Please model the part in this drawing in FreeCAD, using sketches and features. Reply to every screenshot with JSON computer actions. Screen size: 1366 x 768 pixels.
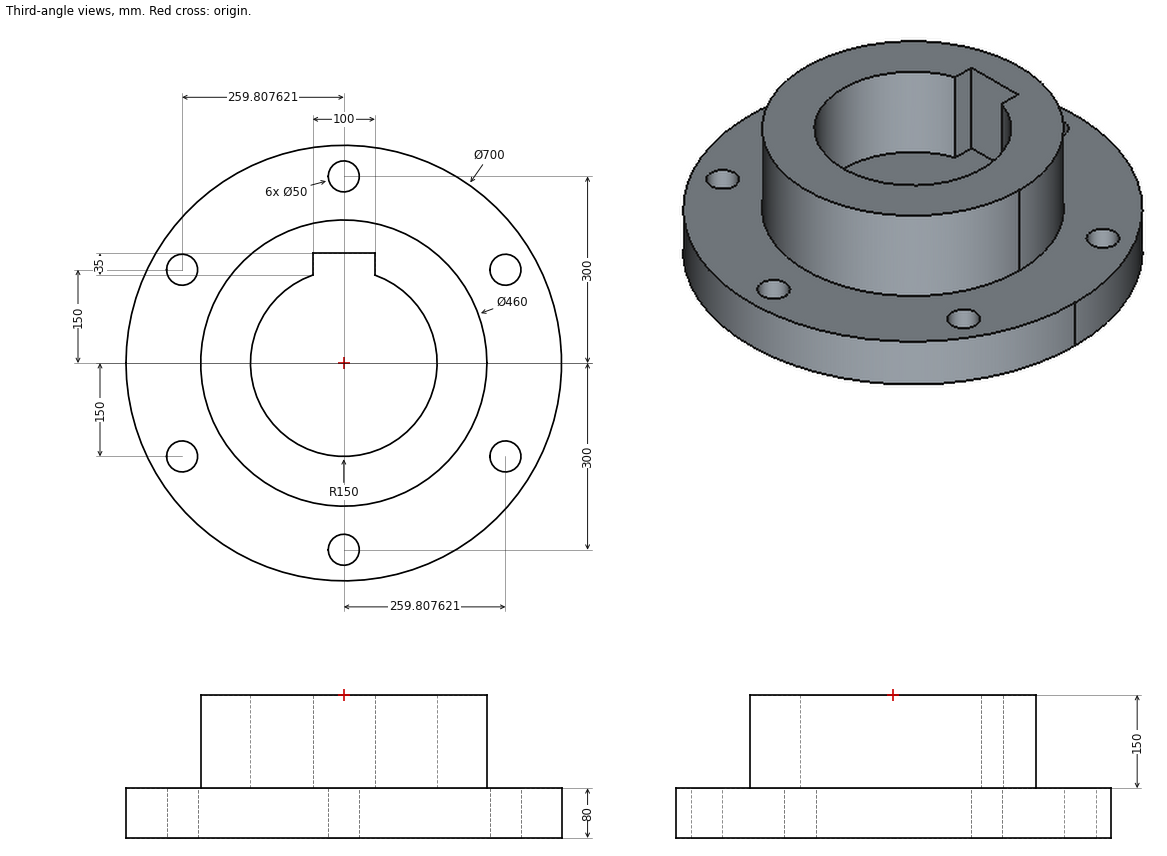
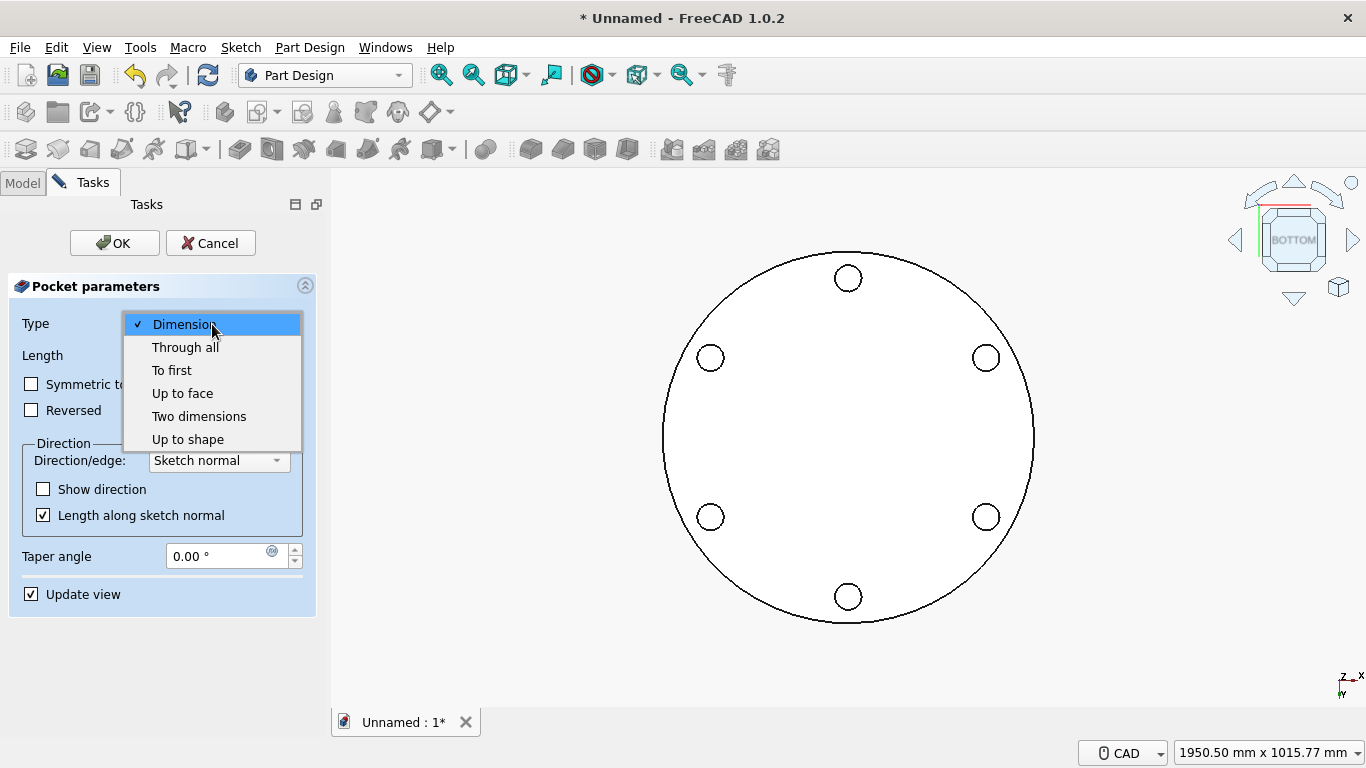
{"action": "left_click", "coordinate": [212, 416]}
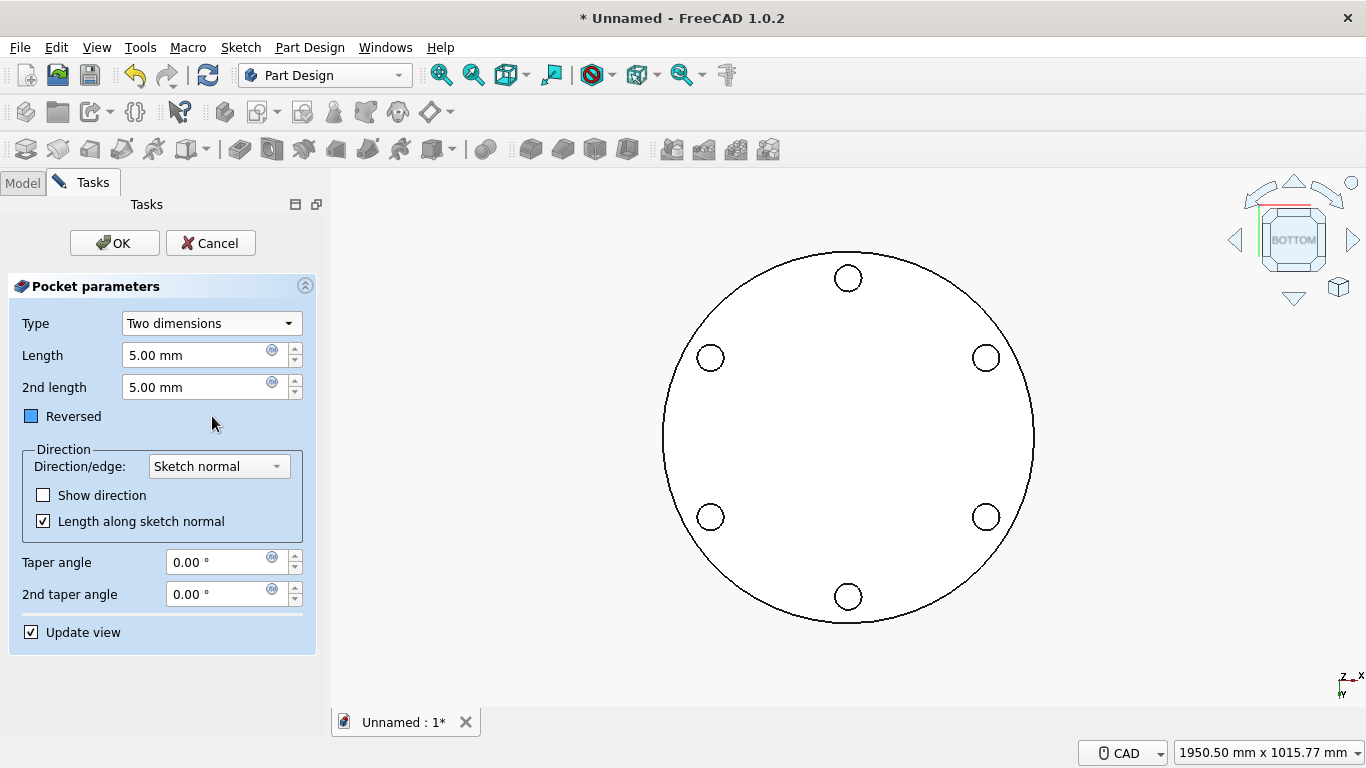
{"action": "triple_click", "coordinate": [204, 355]}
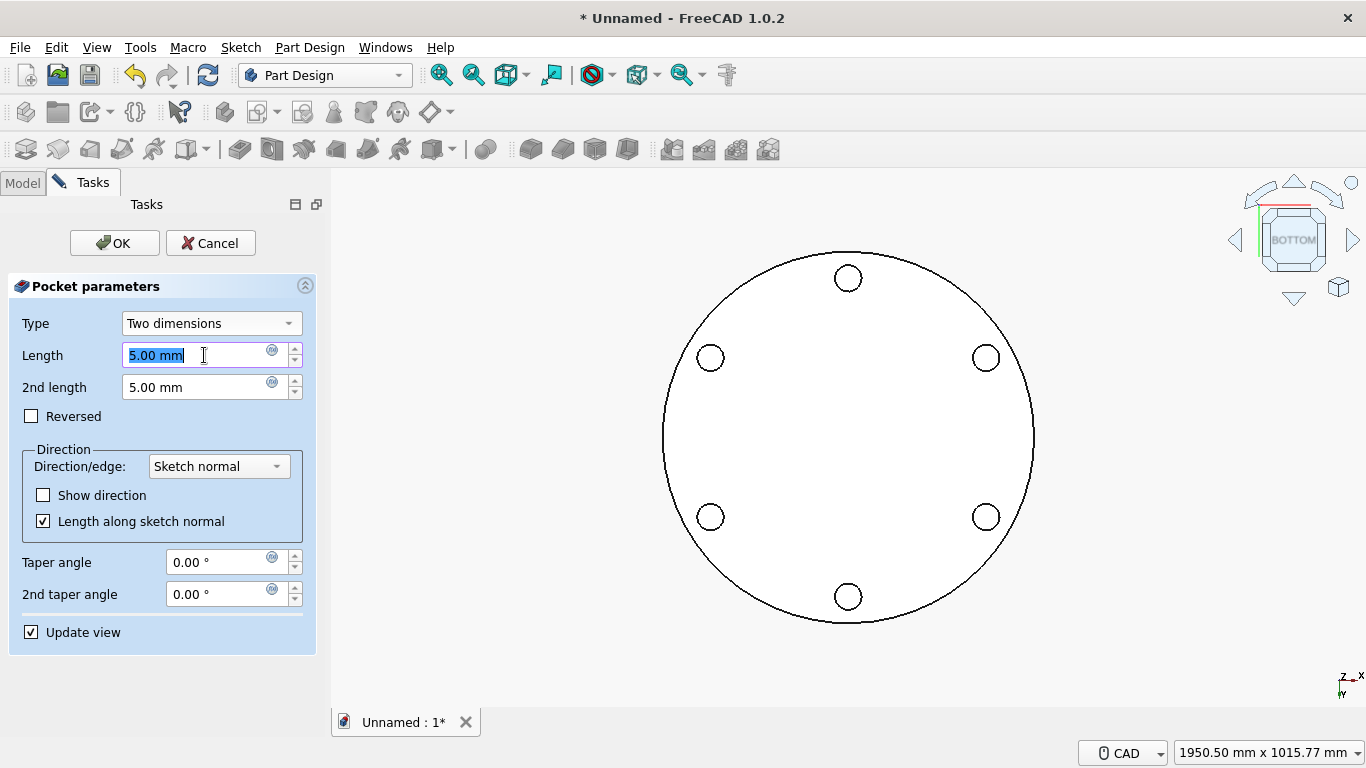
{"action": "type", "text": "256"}
{"action": "key", "text": "Tab"}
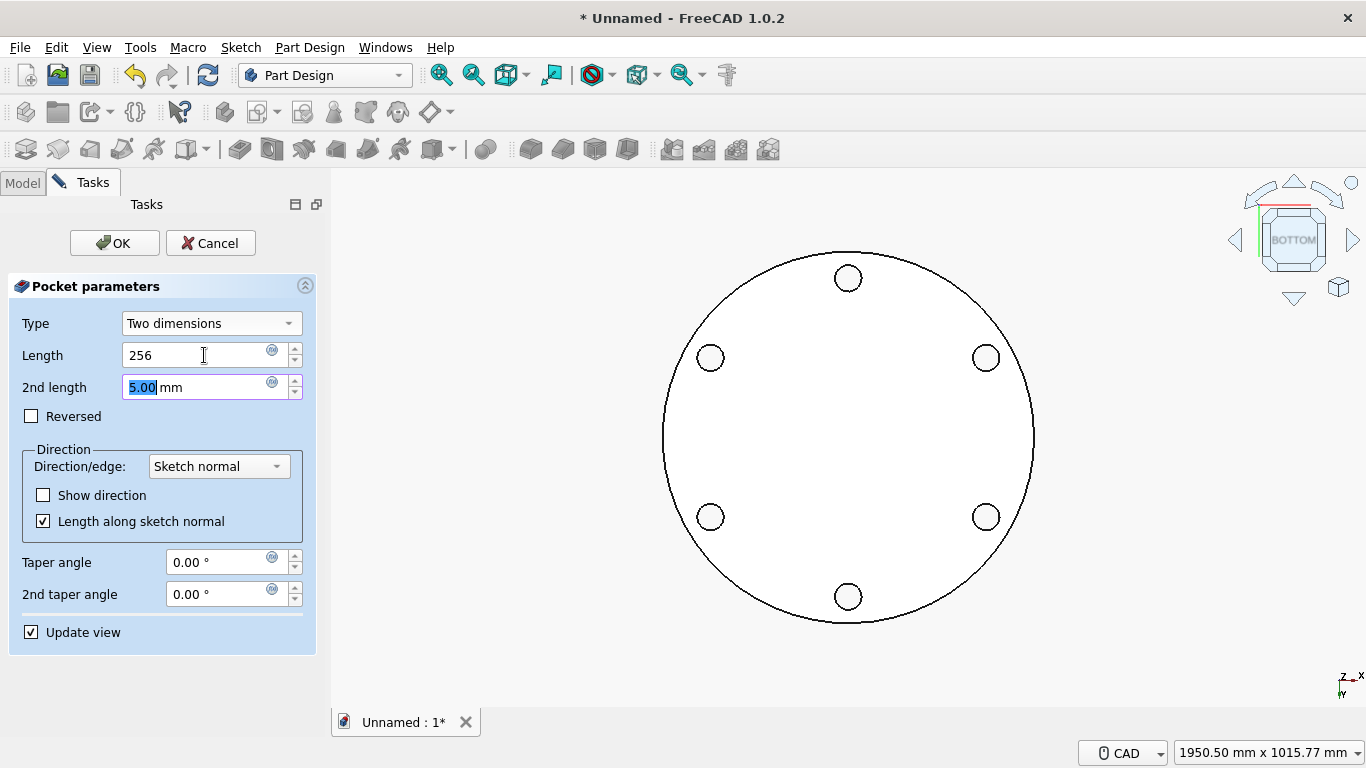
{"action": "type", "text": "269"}
{"action": "key", "text": "Tab"}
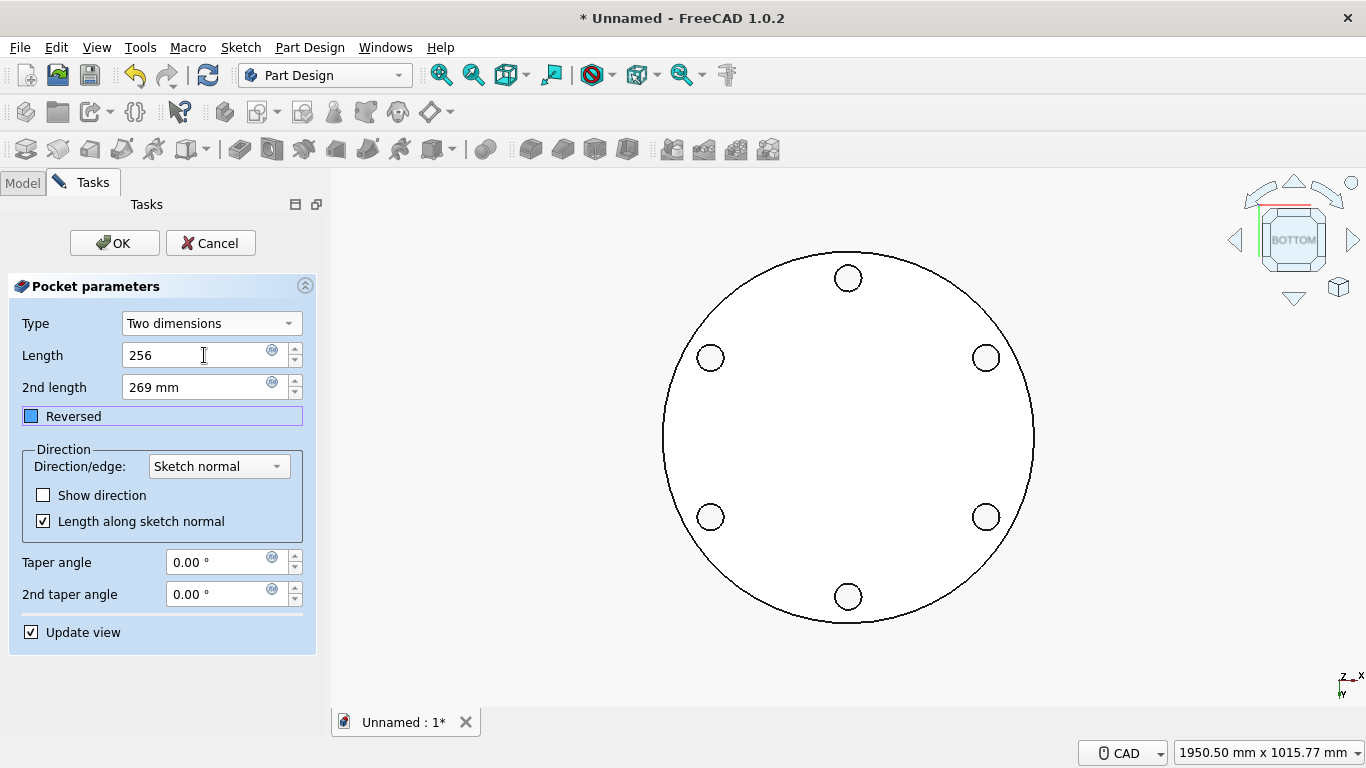
{"action": "left_click", "coordinate": [30, 416]}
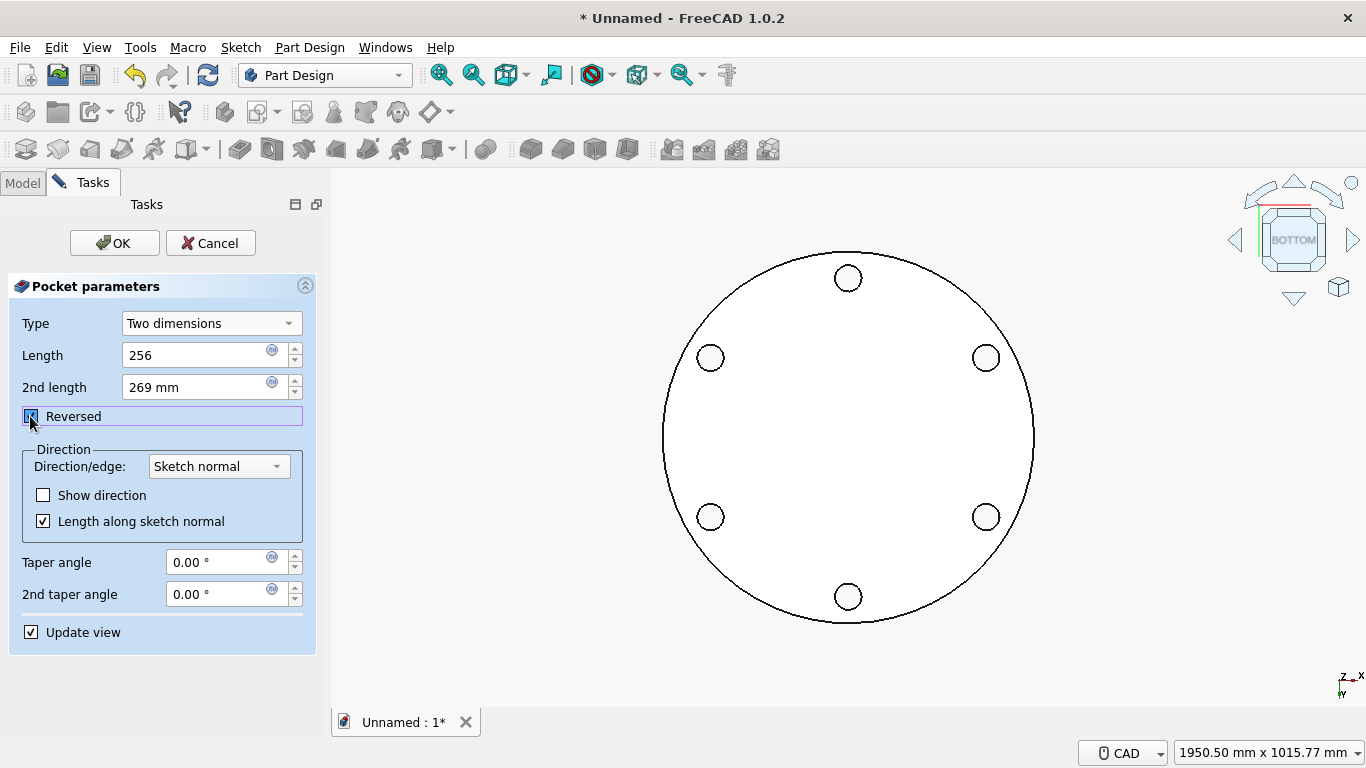
{"action": "left_click", "coordinate": [115, 243]}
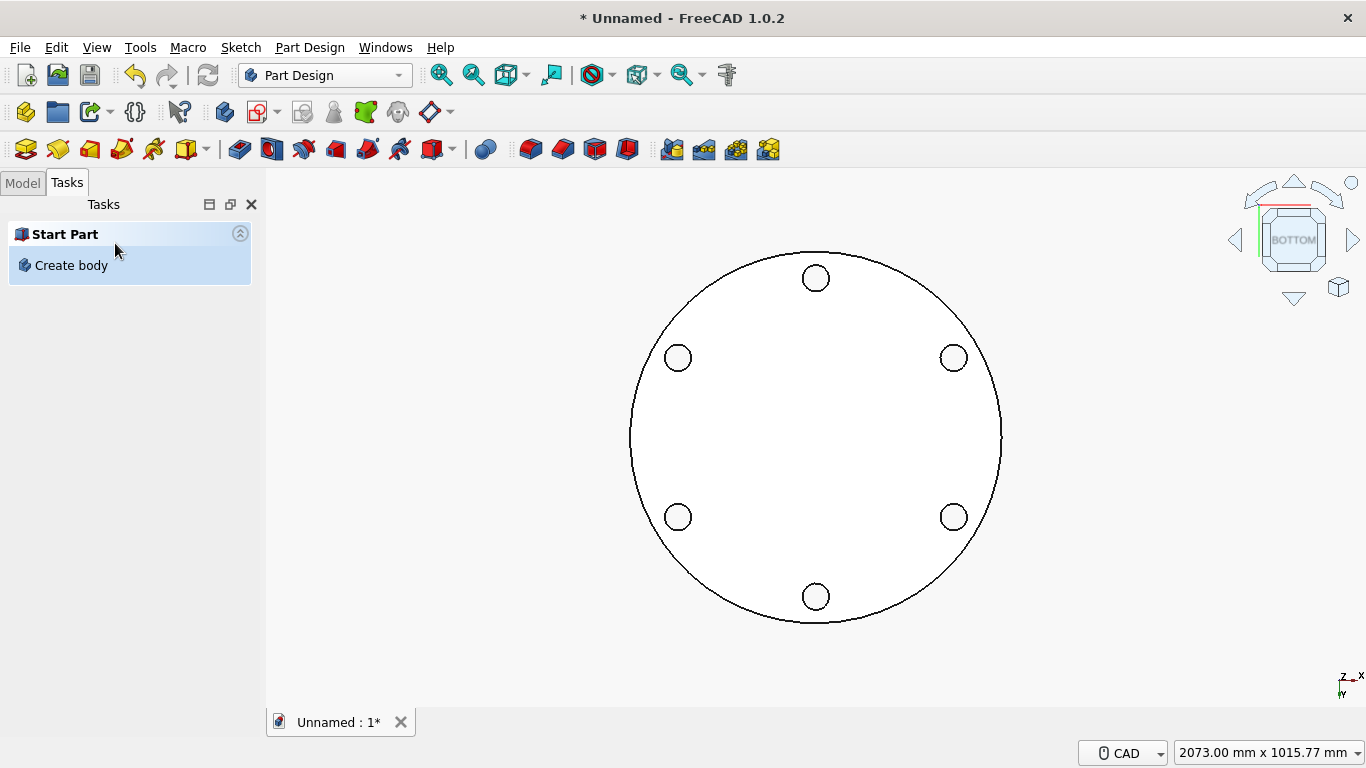
{"action": "key", "text": "0"}